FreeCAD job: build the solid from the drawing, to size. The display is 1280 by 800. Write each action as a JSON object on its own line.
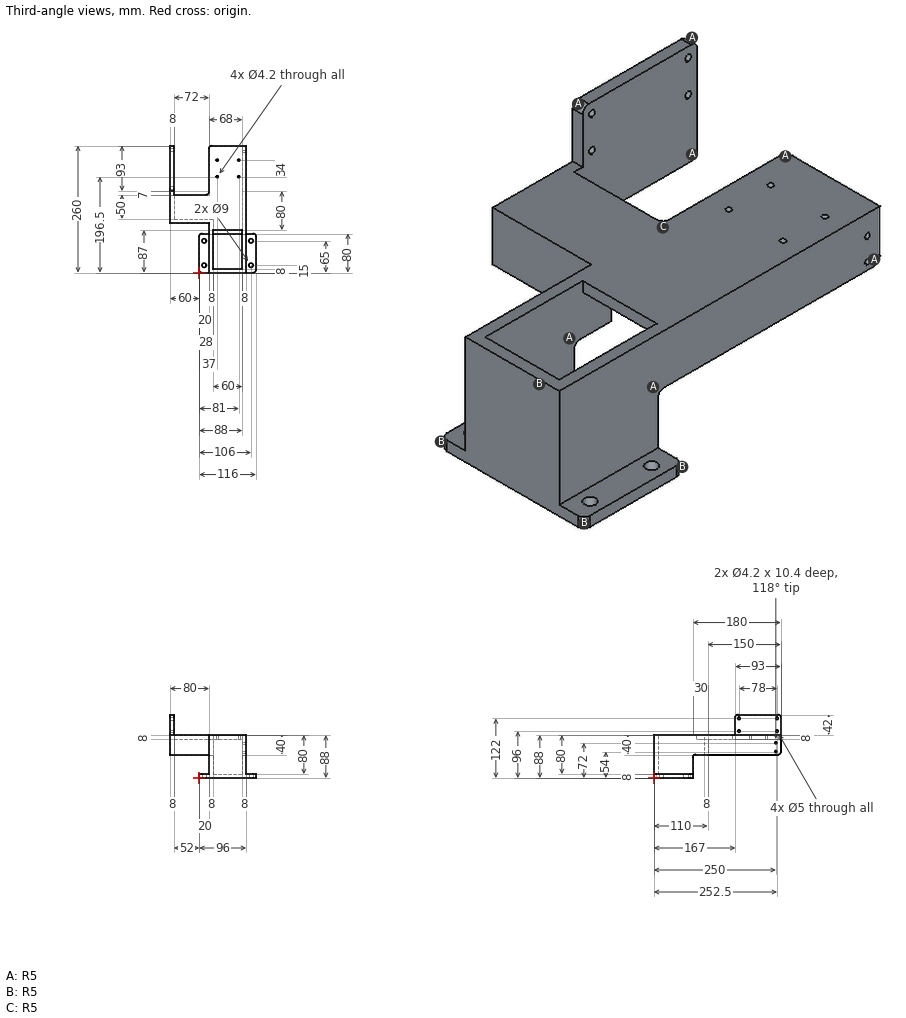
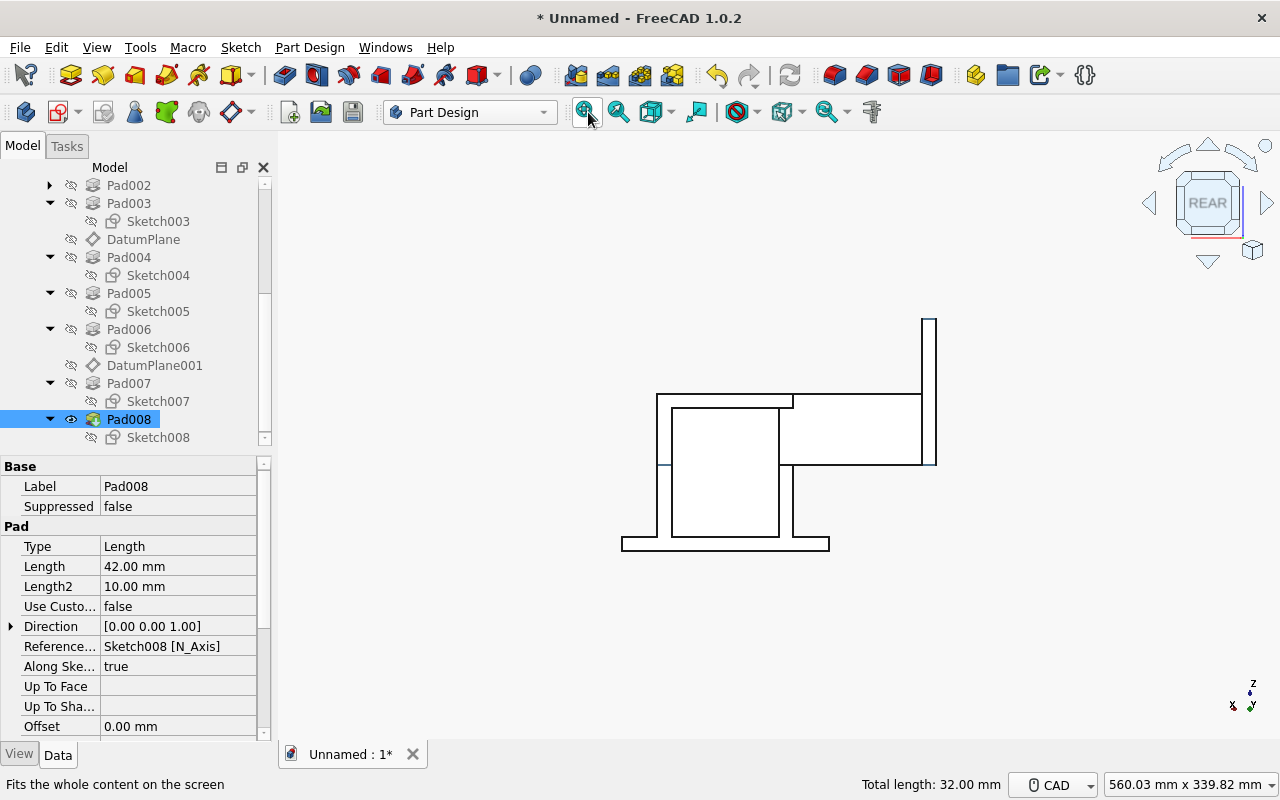
{"action": "left_click", "coordinate": [588, 112]}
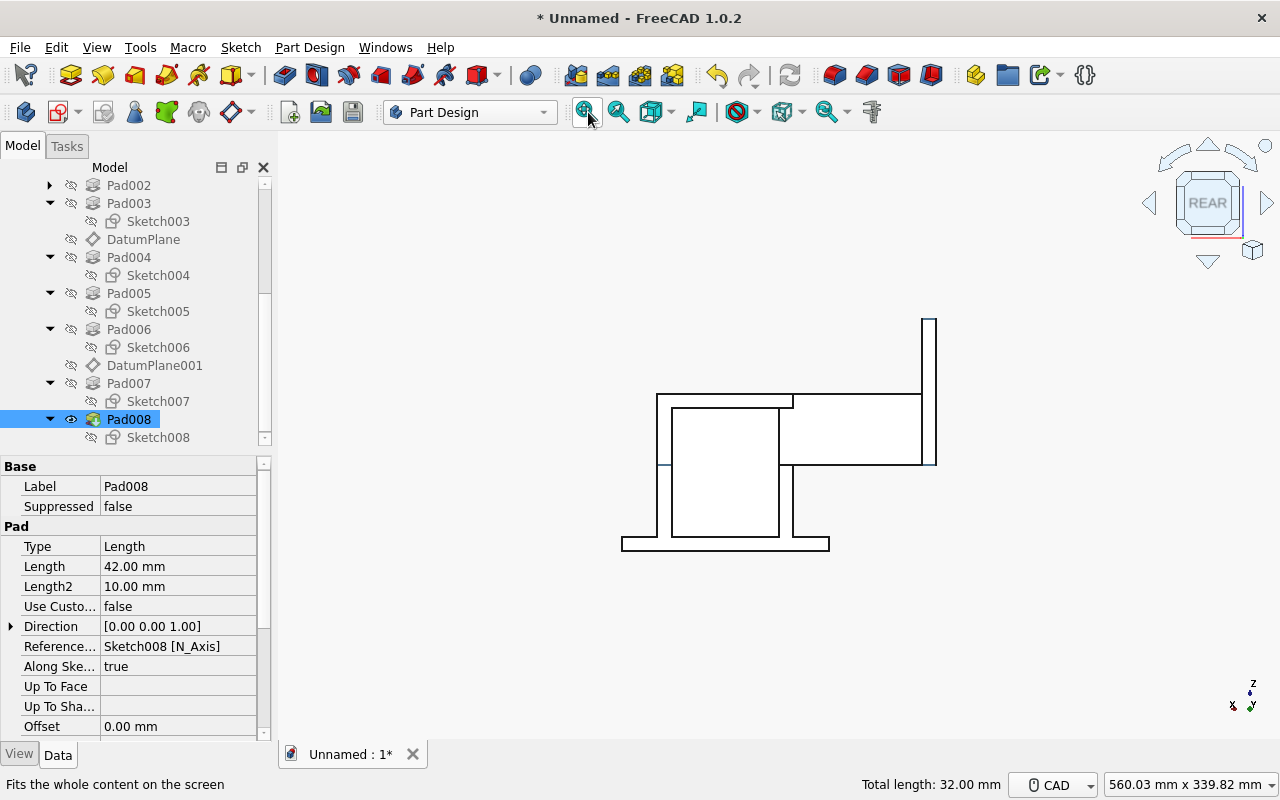
{"action": "left_click", "coordinate": [793, 400], "text": "ctrl"}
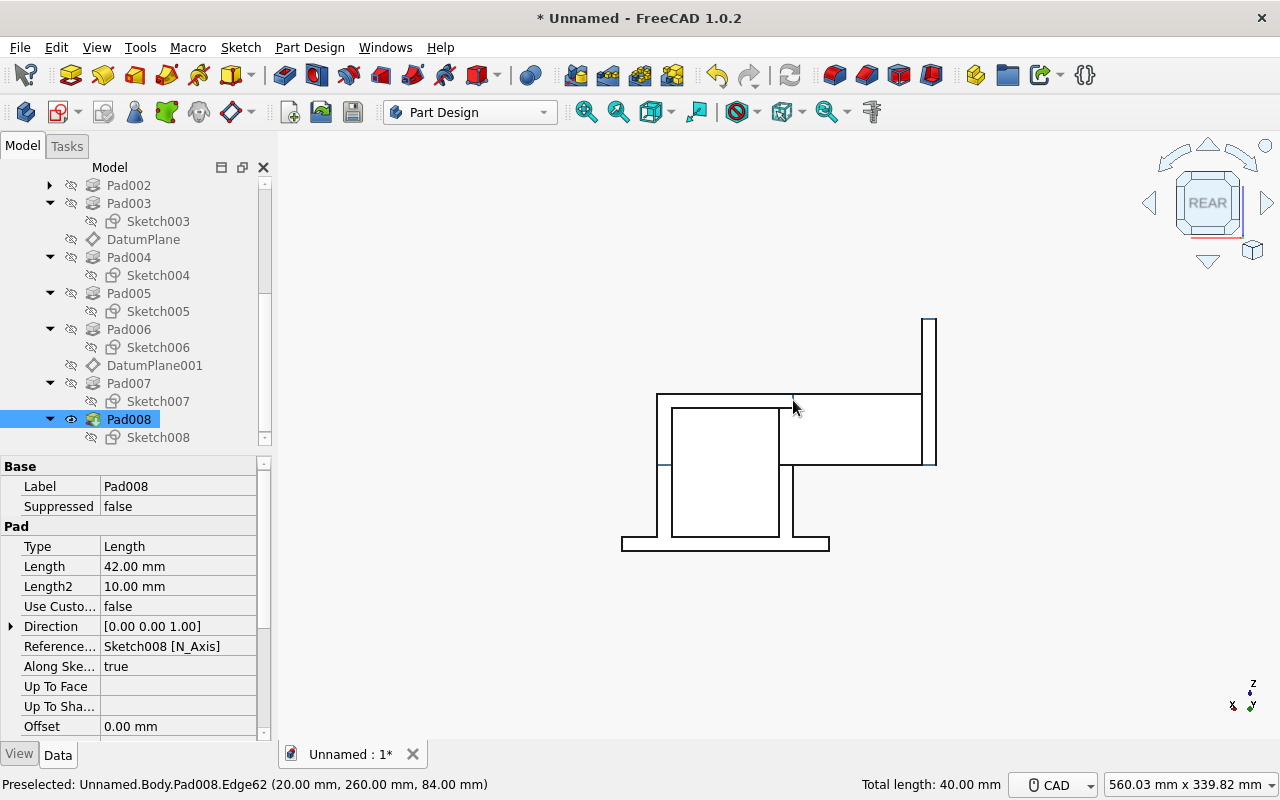
{"action": "scroll", "coordinate": [786, 464], "scroll_direction": "up", "scroll_amount": 6}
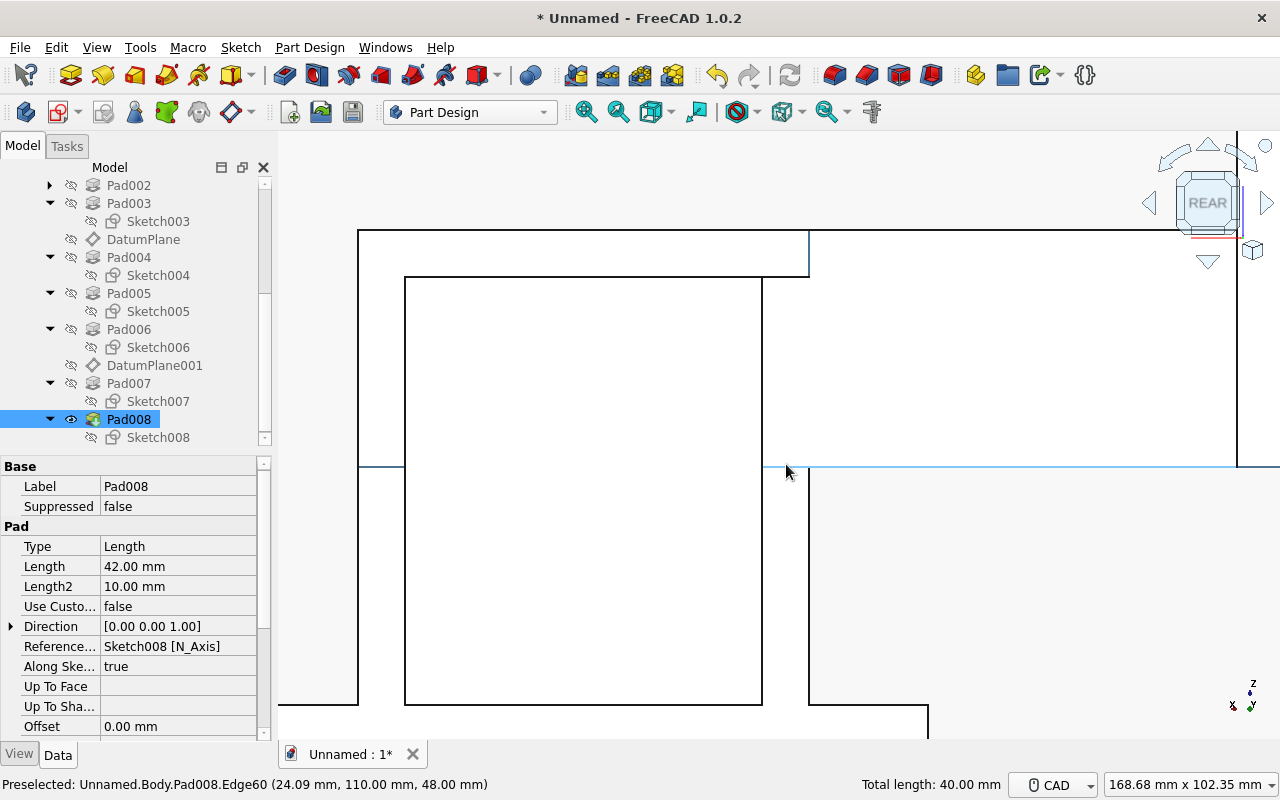
{"action": "left_click", "coordinate": [588, 112]}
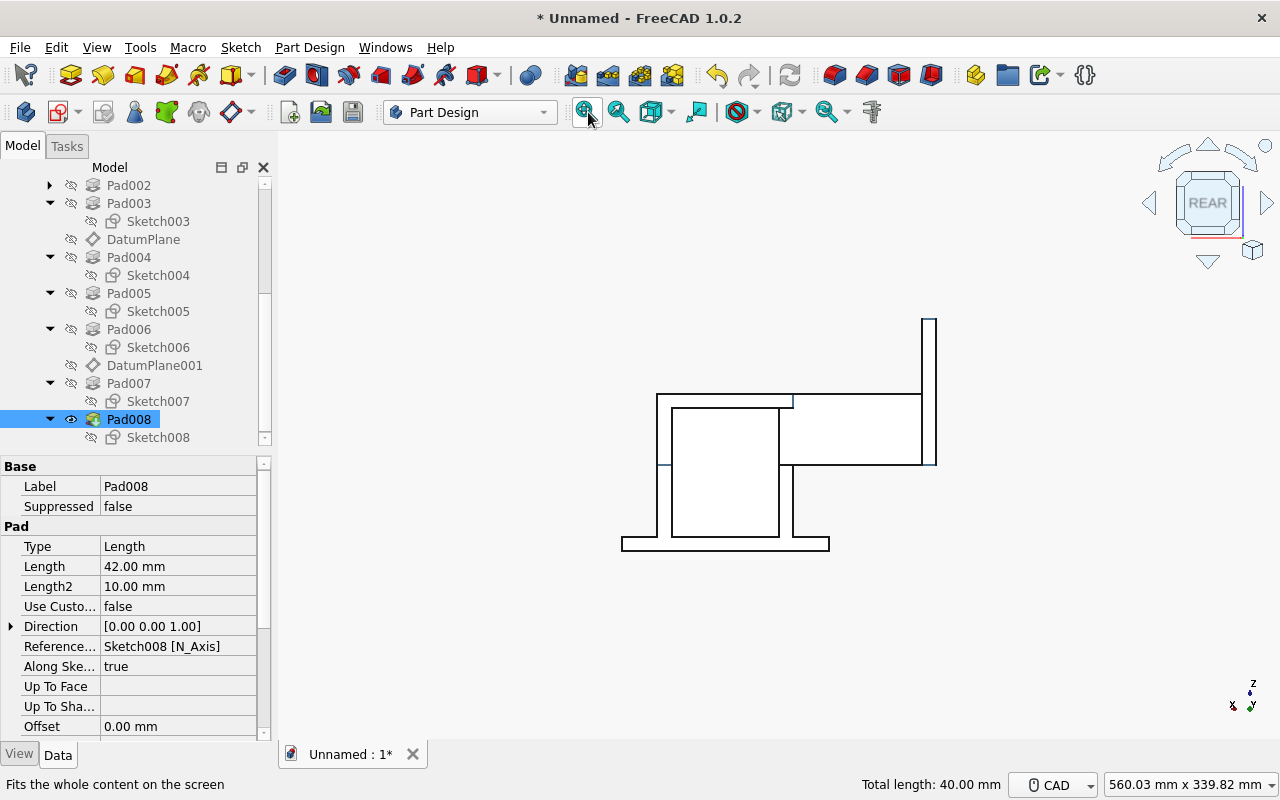
{"action": "key", "text": "6"}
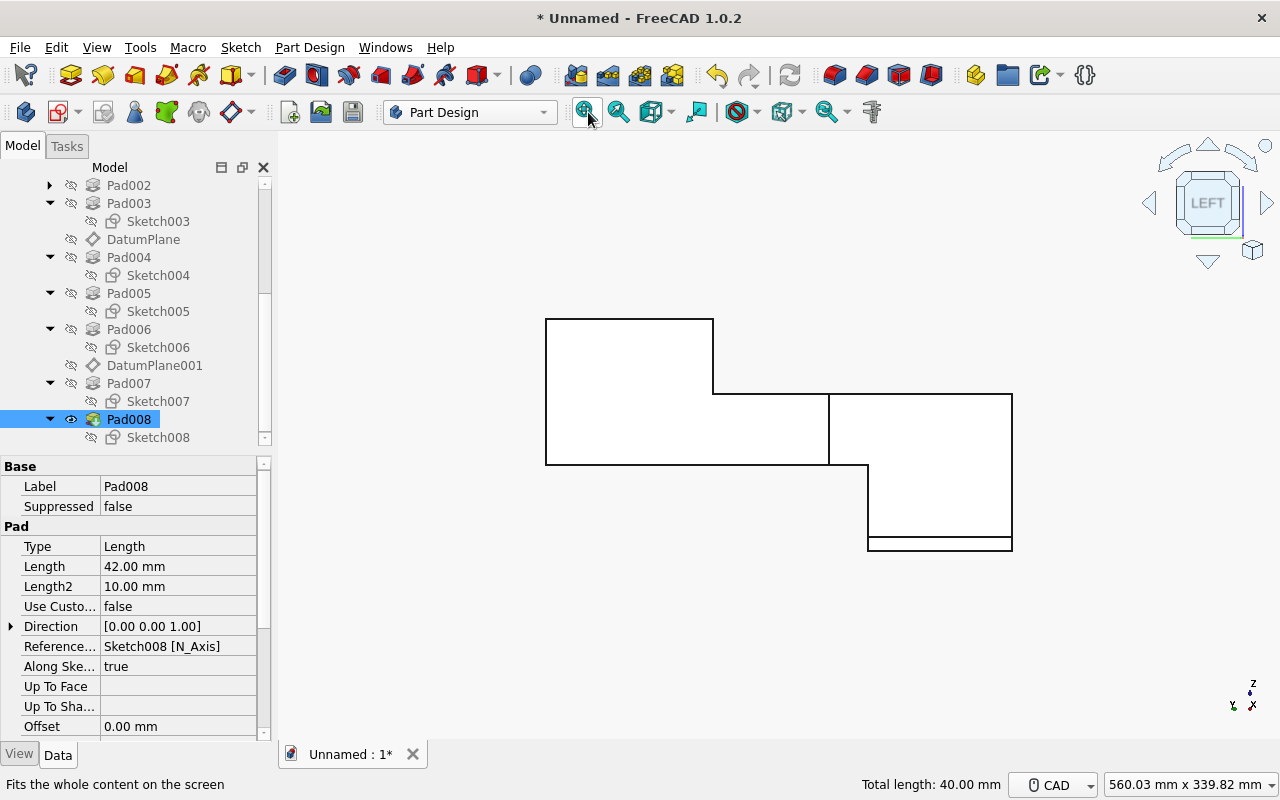
{"action": "scroll", "coordinate": [868, 464], "scroll_direction": "up", "scroll_amount": 6}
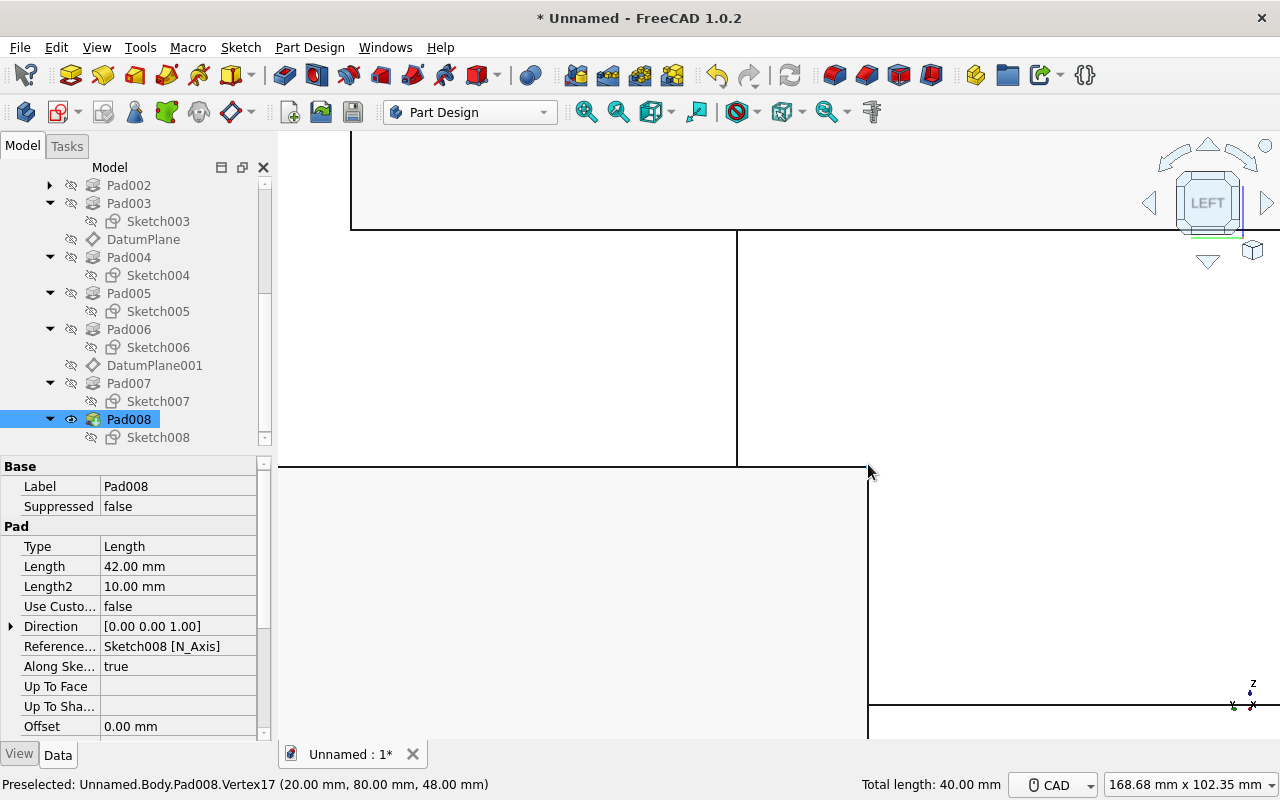
{"action": "left_click", "coordinate": [588, 112]}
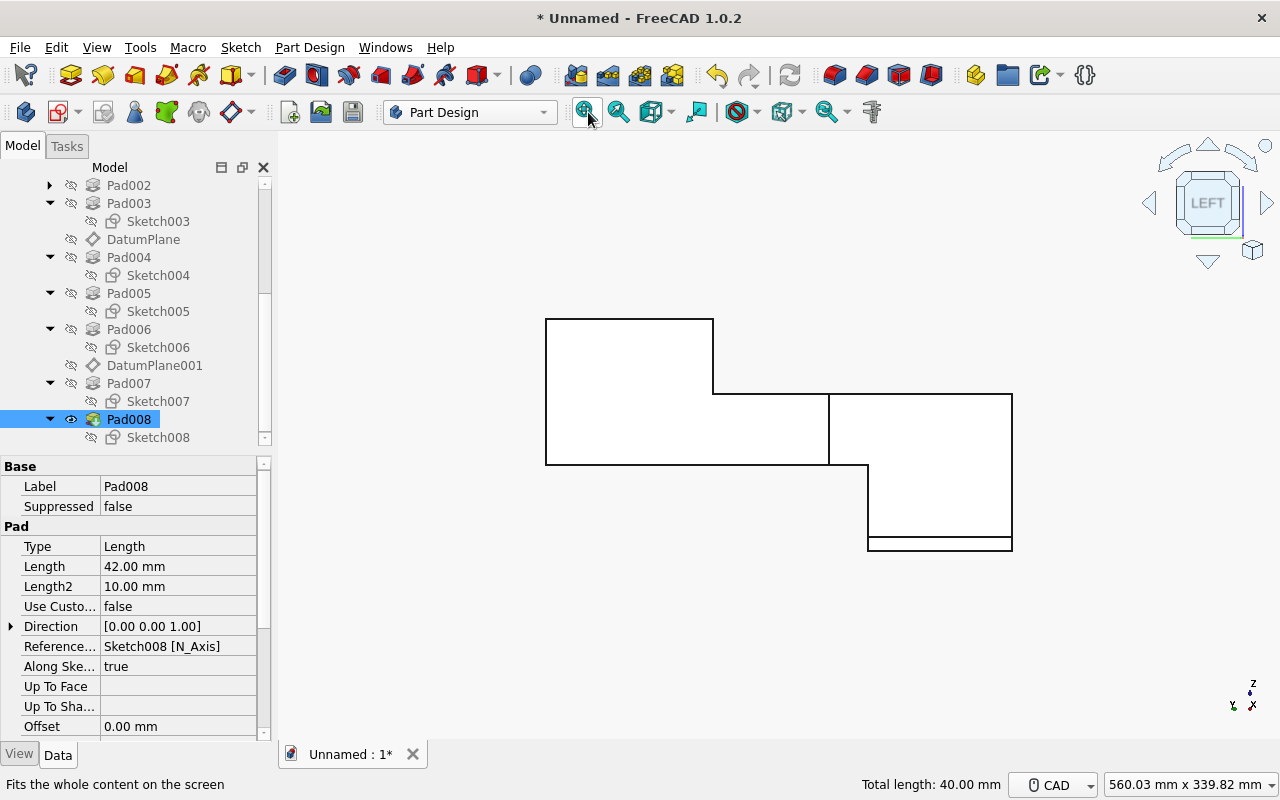
{"action": "key", "text": "v 3"}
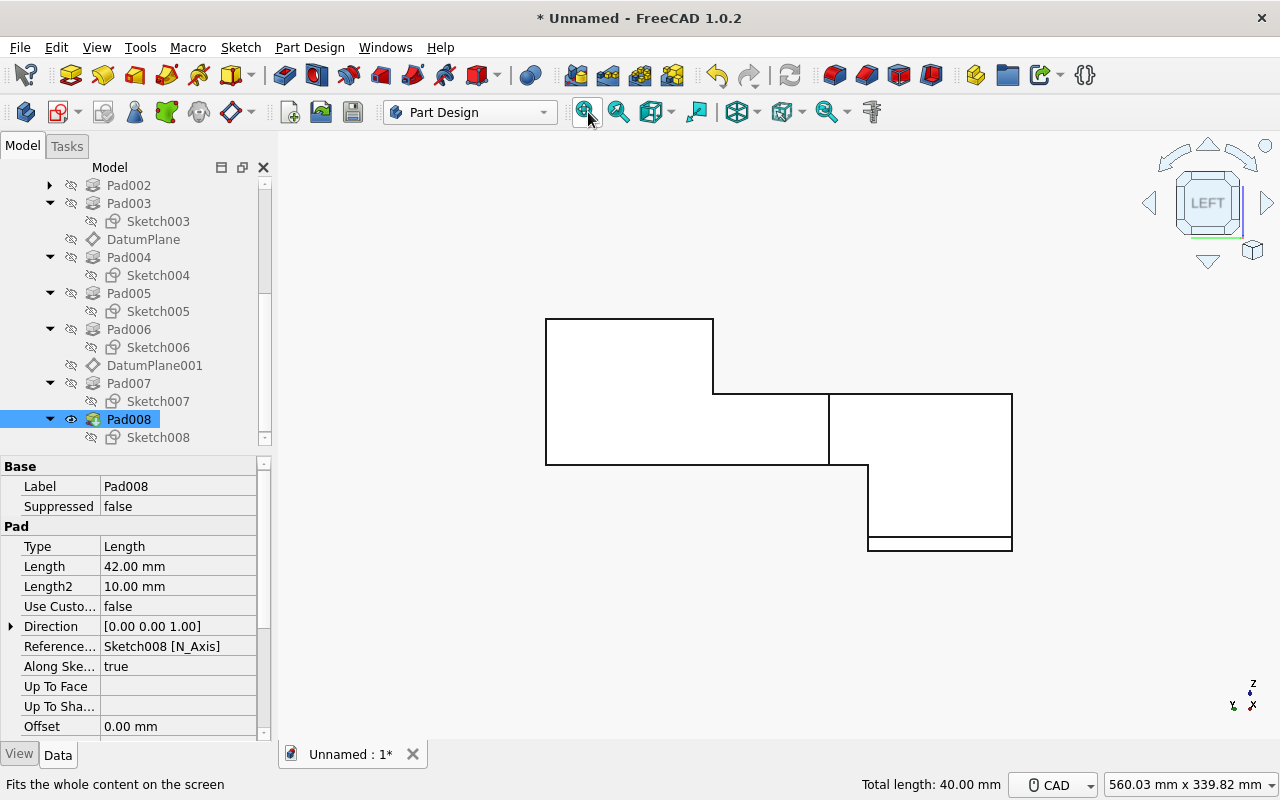
{"action": "key", "text": "0"}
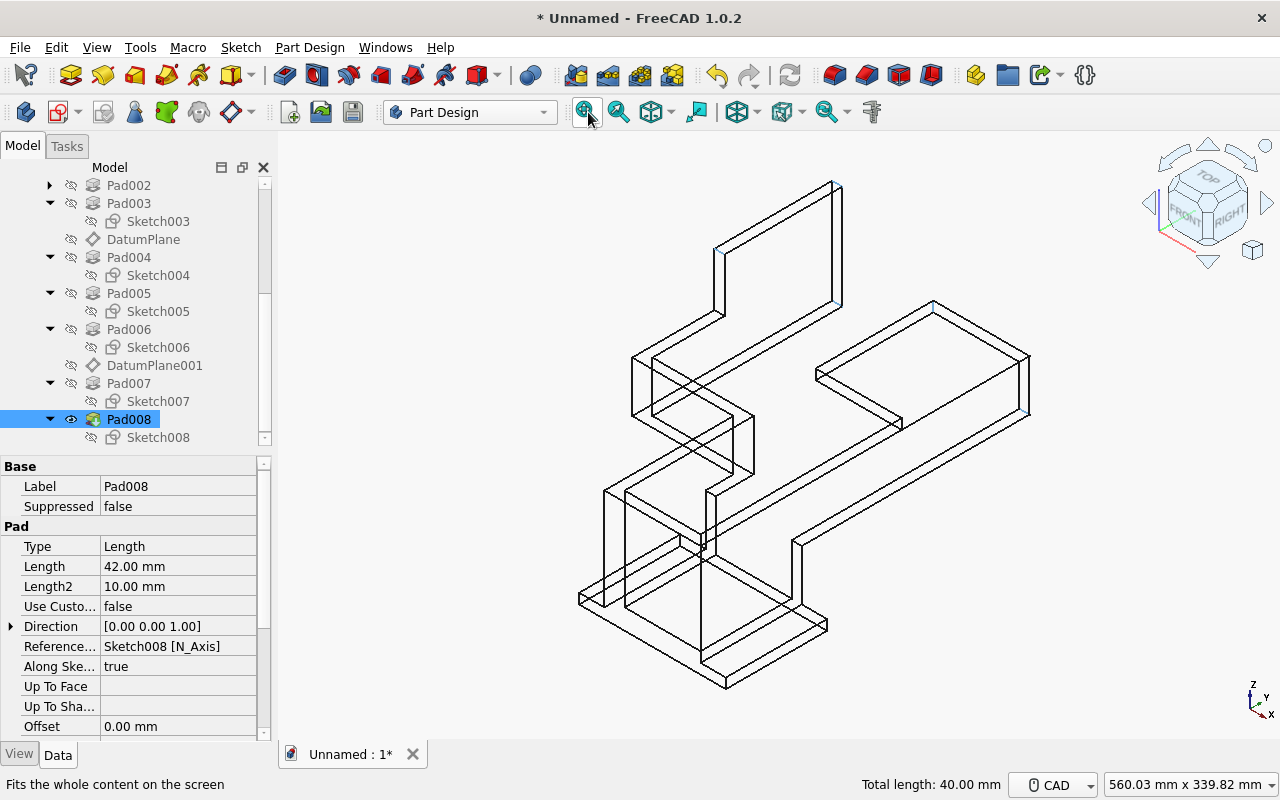
{"action": "left_click", "coordinate": [710, 492], "text": "ctrl"}